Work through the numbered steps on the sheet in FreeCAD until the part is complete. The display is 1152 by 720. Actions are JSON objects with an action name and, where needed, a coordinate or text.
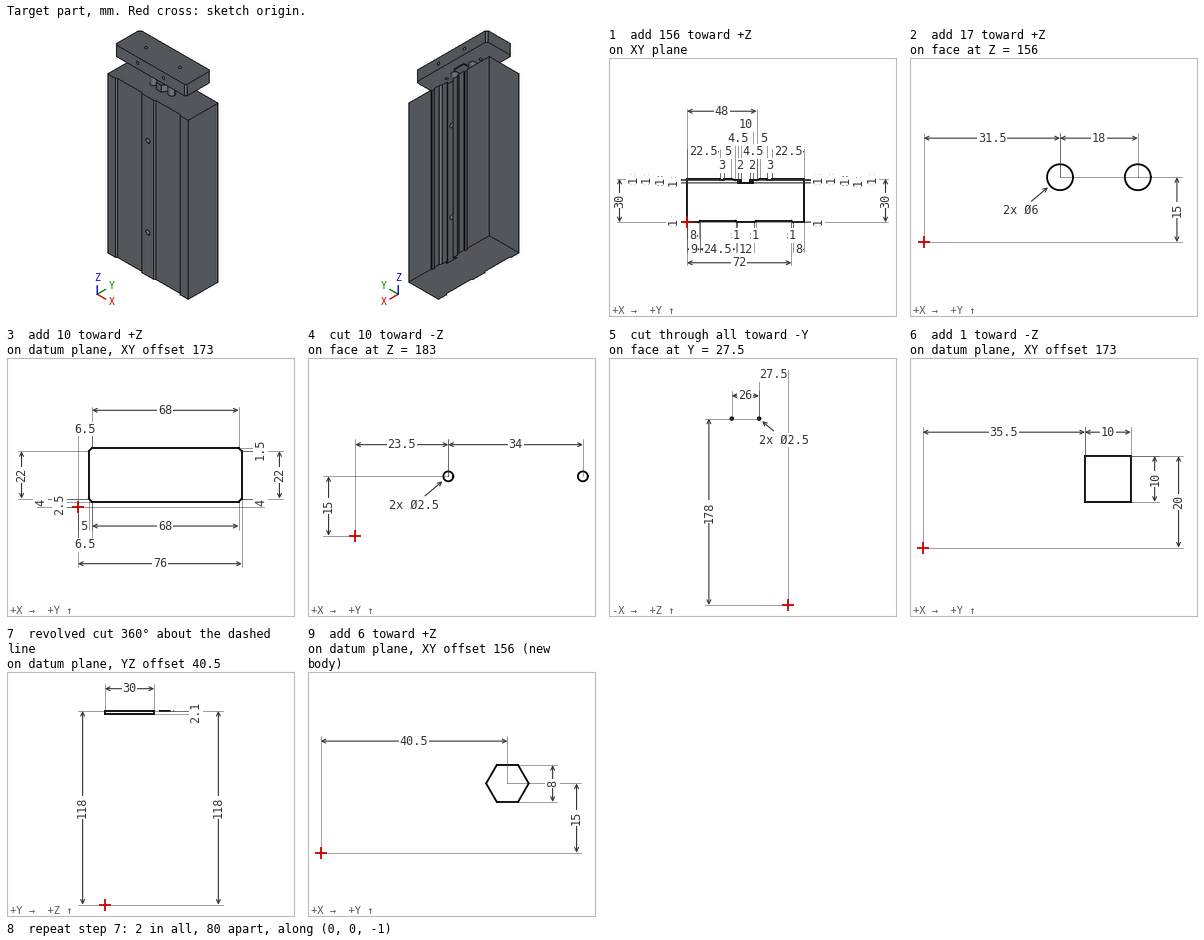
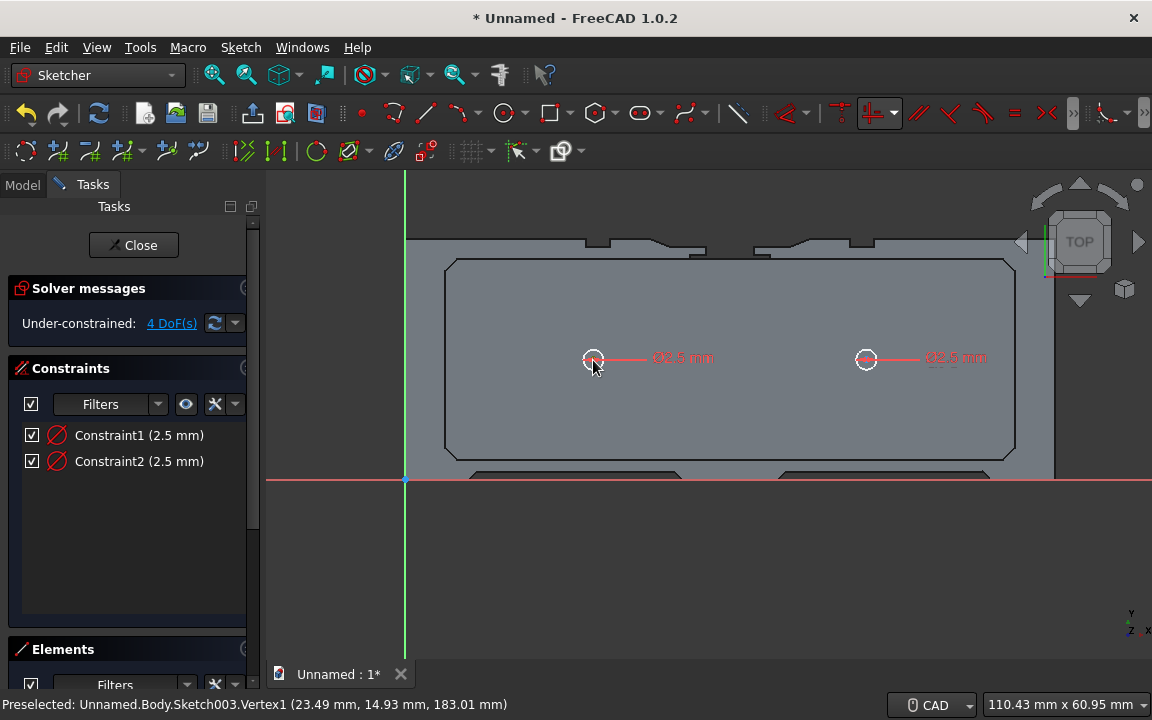
{"action": "left_click", "coordinate": [866, 360]}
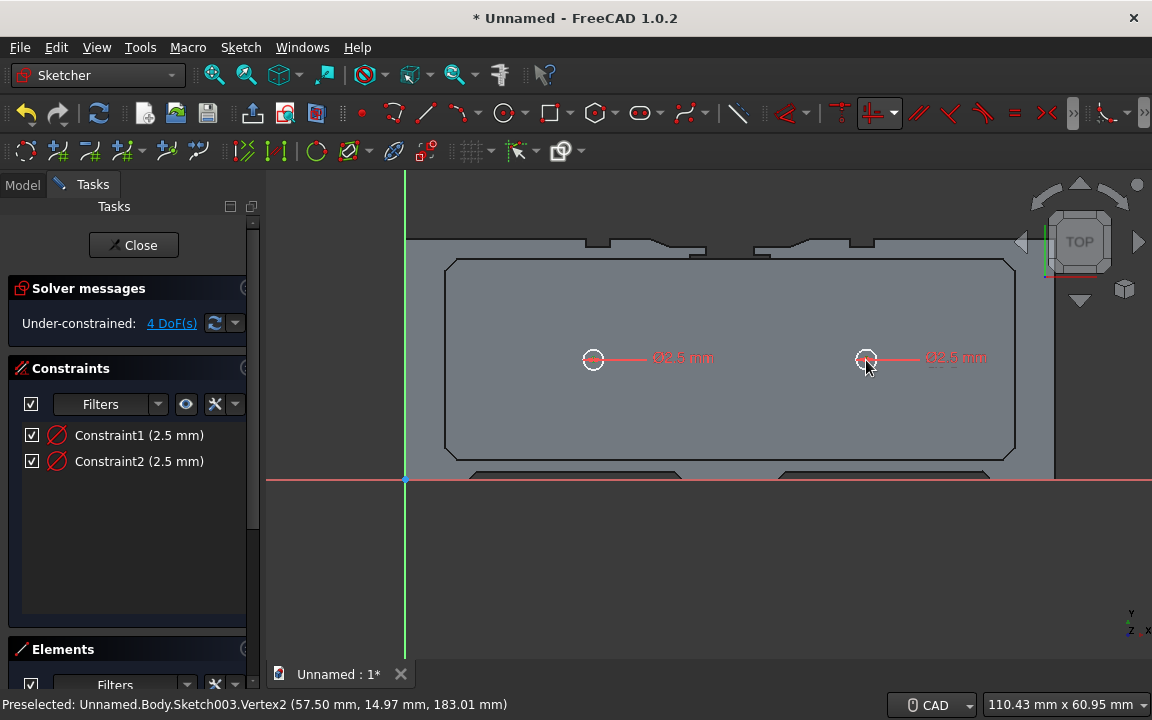
{"action": "key", "text": "h"}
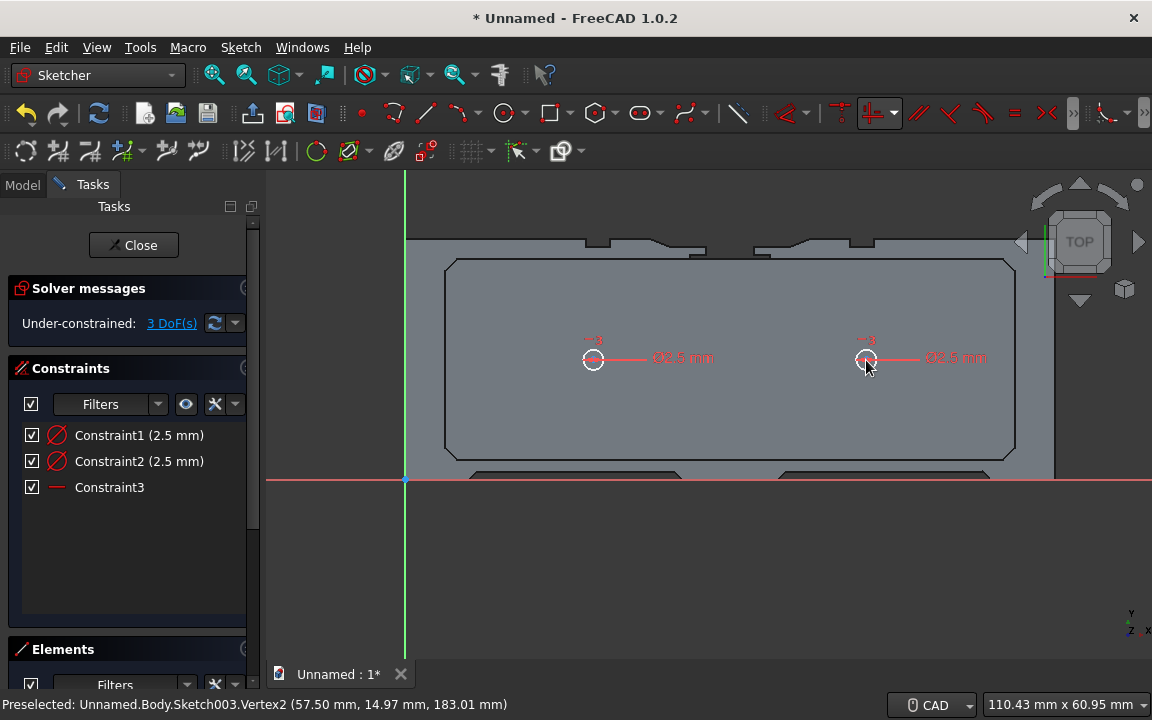
{"action": "key", "text": "d"}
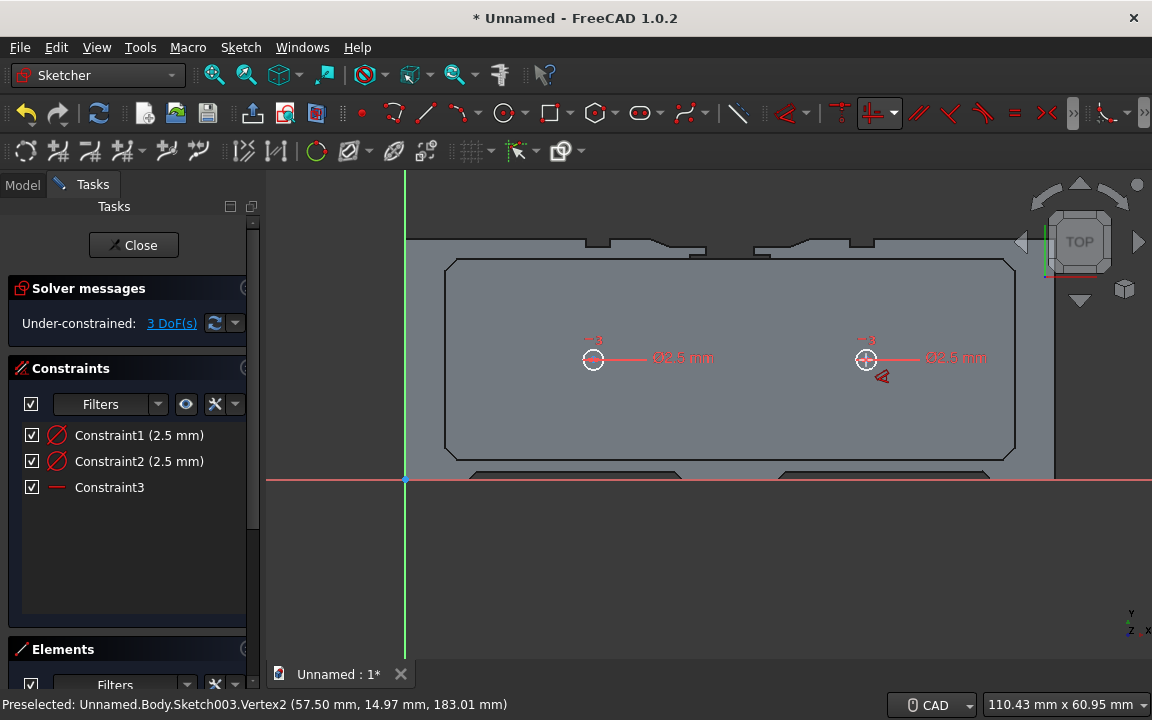
{"action": "left_click", "coordinate": [593, 360]}
{"action": "left_click", "coordinate": [371, 420]}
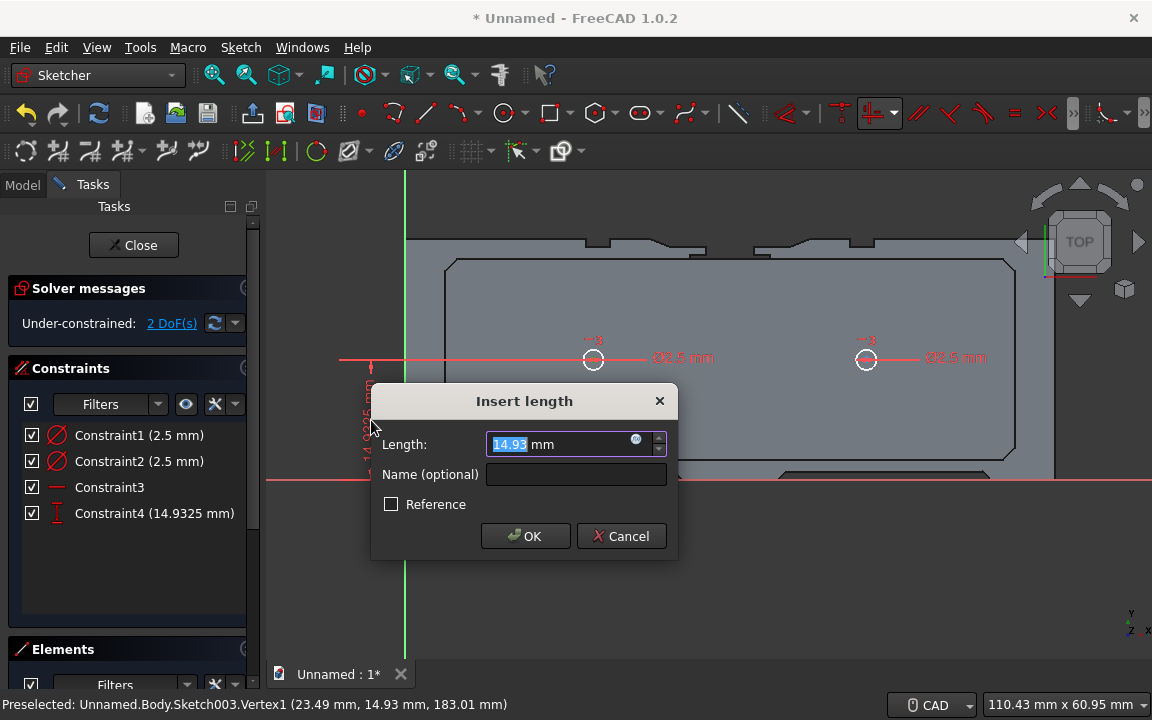
{"action": "type", "text": "15"}
{"action": "key", "text": "Return"}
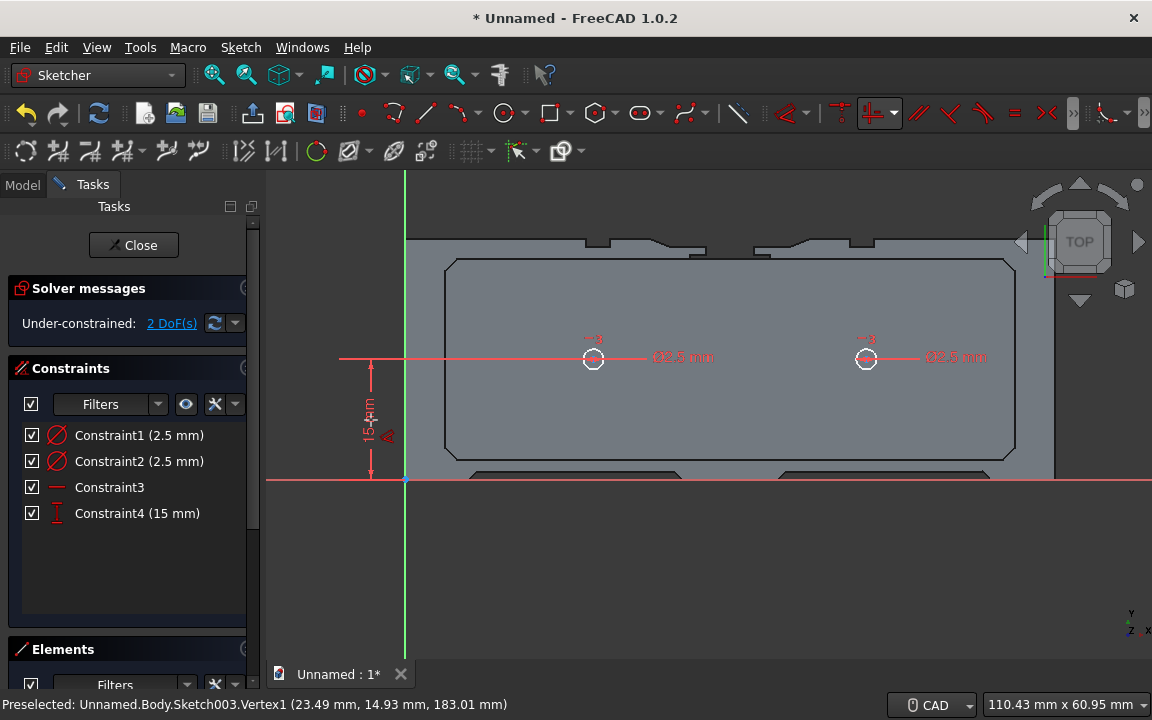
{"action": "left_click", "coordinate": [593, 359]}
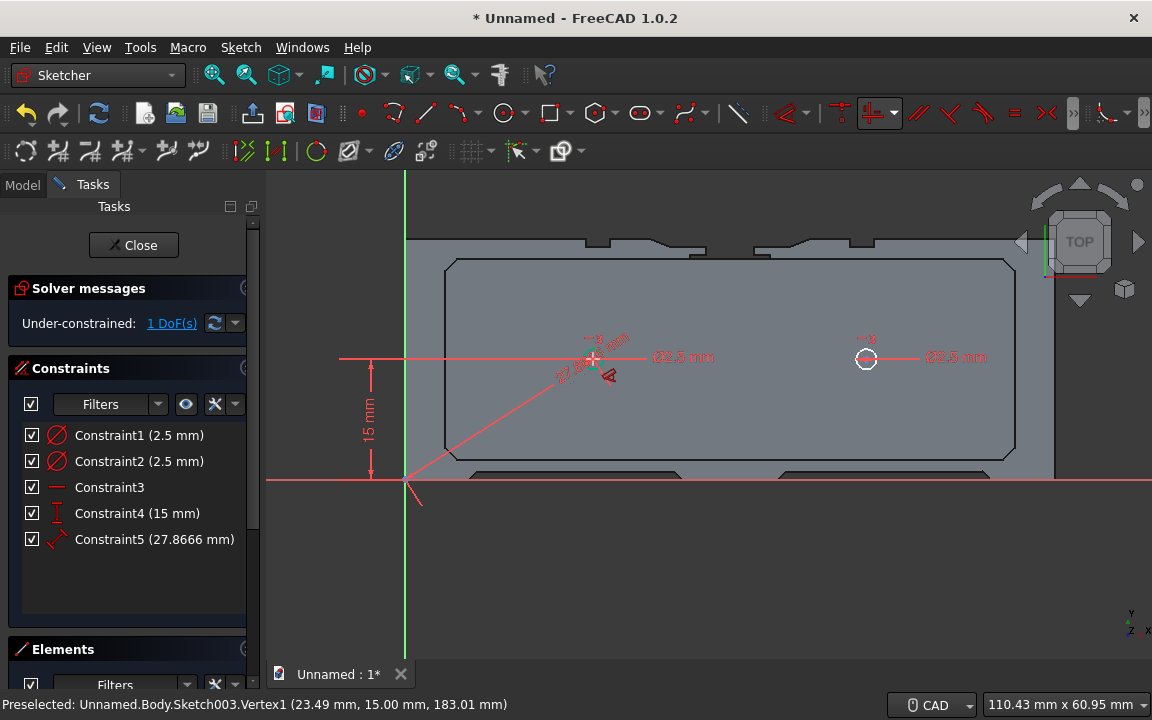
{"action": "left_click", "coordinate": [866, 359]}
{"action": "left_click", "coordinate": [730, 325]}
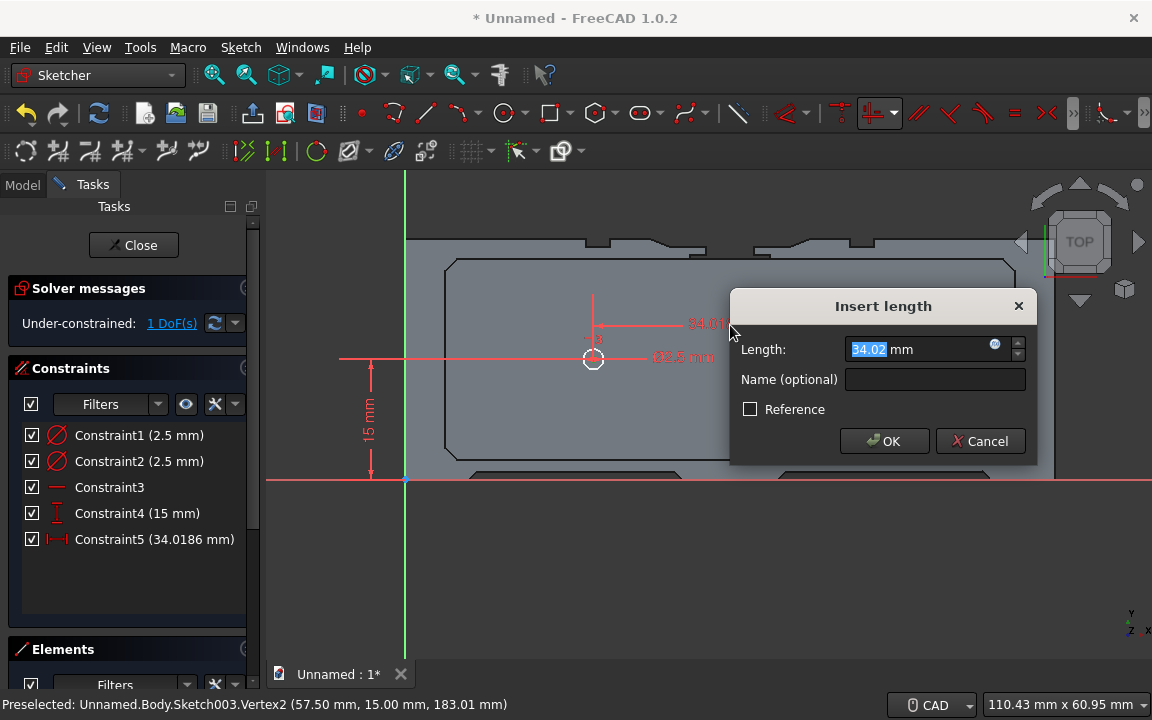
{"action": "type", "text": "34"}
{"action": "key", "text": "Return"}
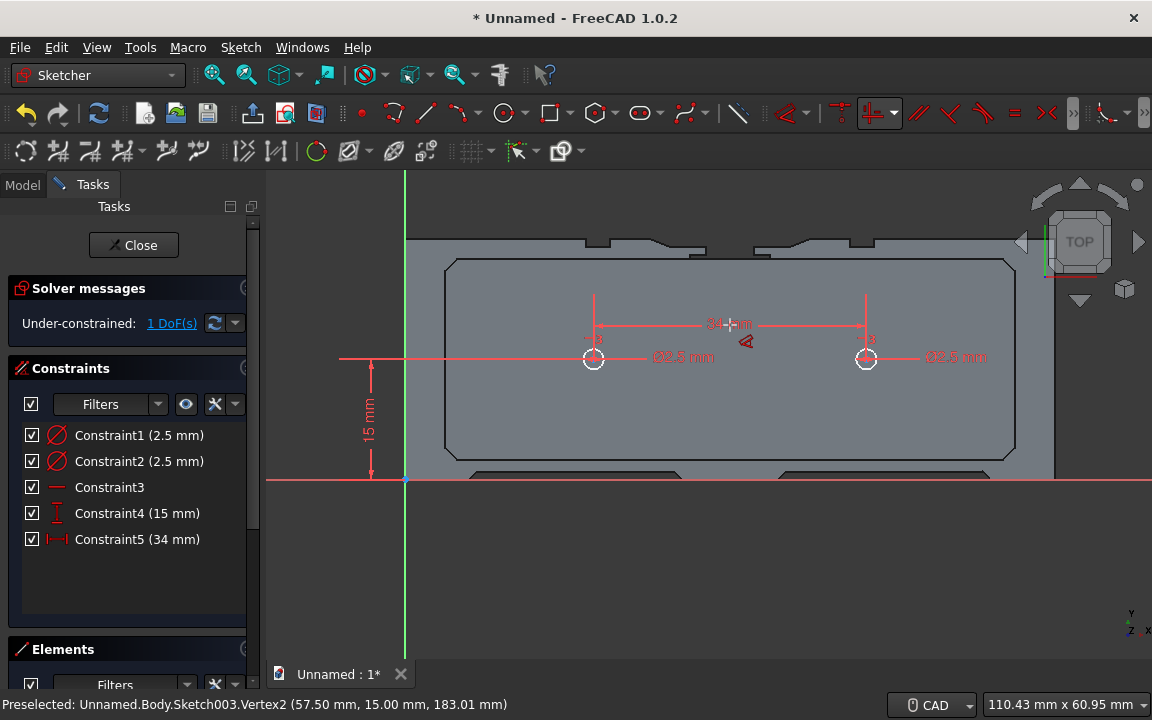
{"action": "left_click", "coordinate": [594, 359]}
{"action": "left_click", "coordinate": [499, 514]}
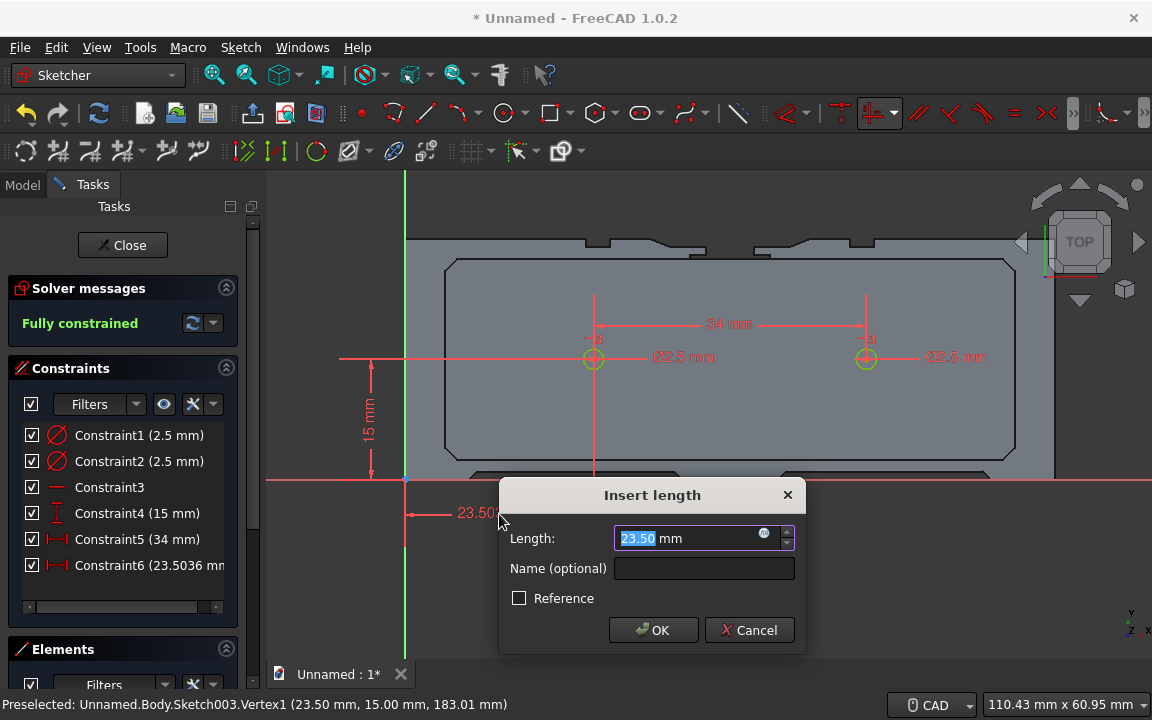
{"action": "type", "text": "23.5"}
{"action": "key", "text": "Return"}
{"action": "key", "text": "Escape"}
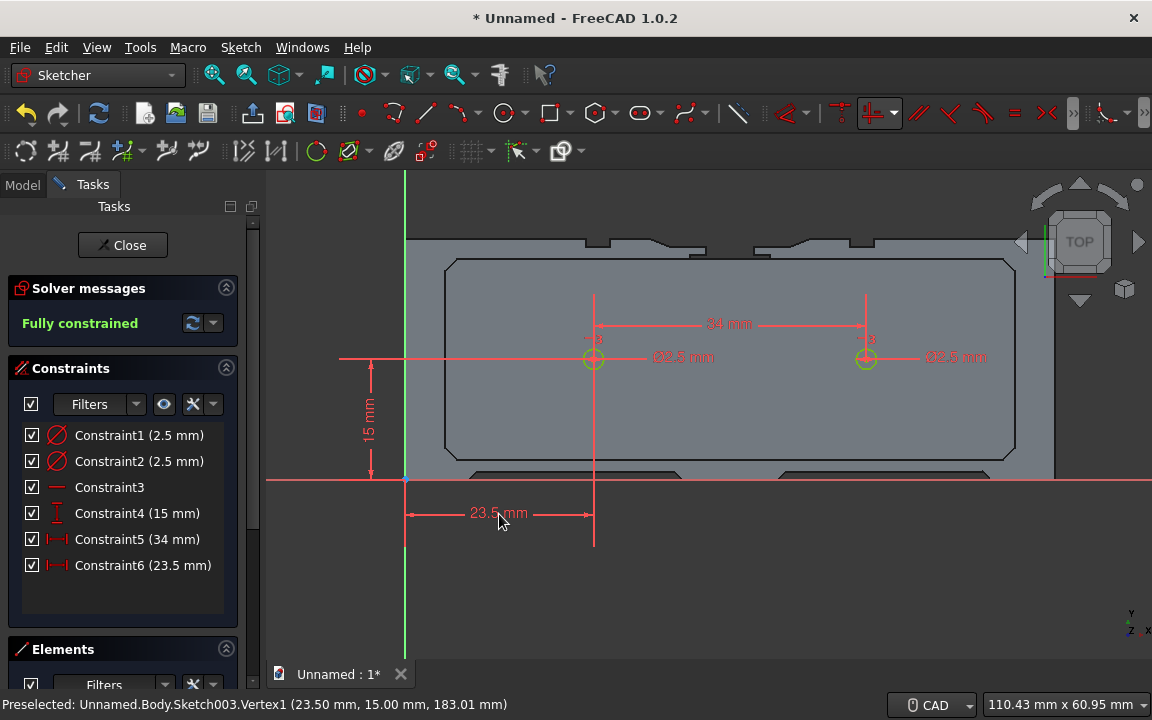
{"action": "left_click", "coordinate": [123, 245]}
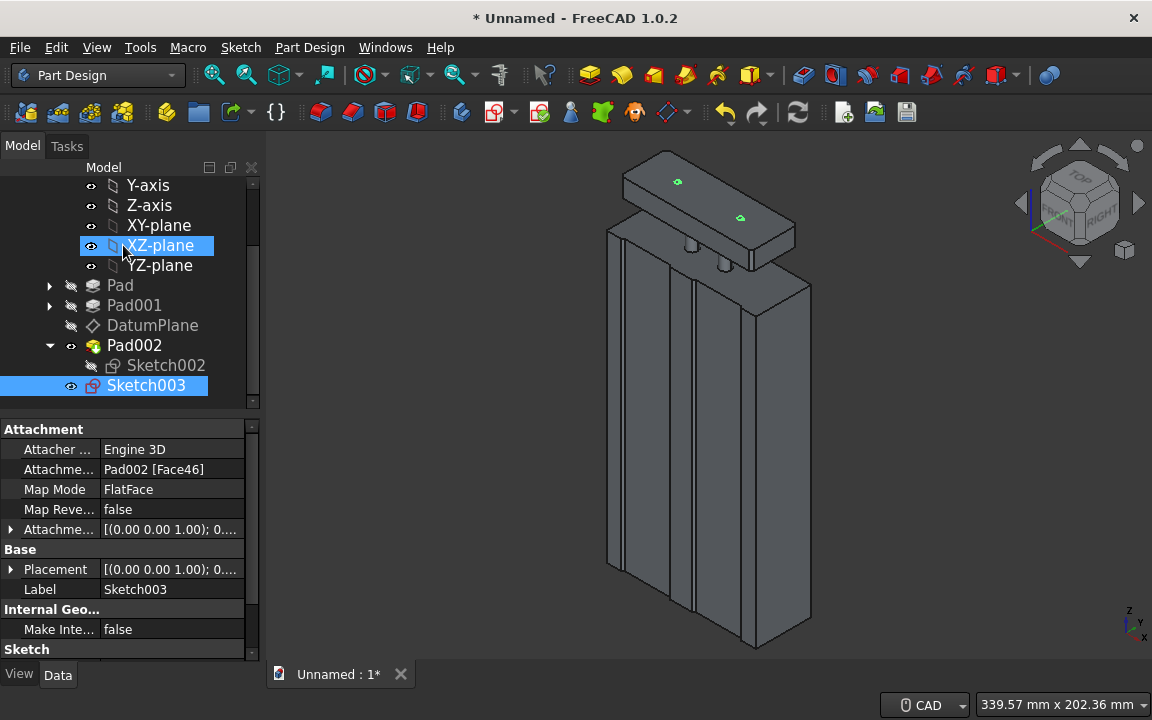
{"action": "left_click", "coordinate": [804, 76]}